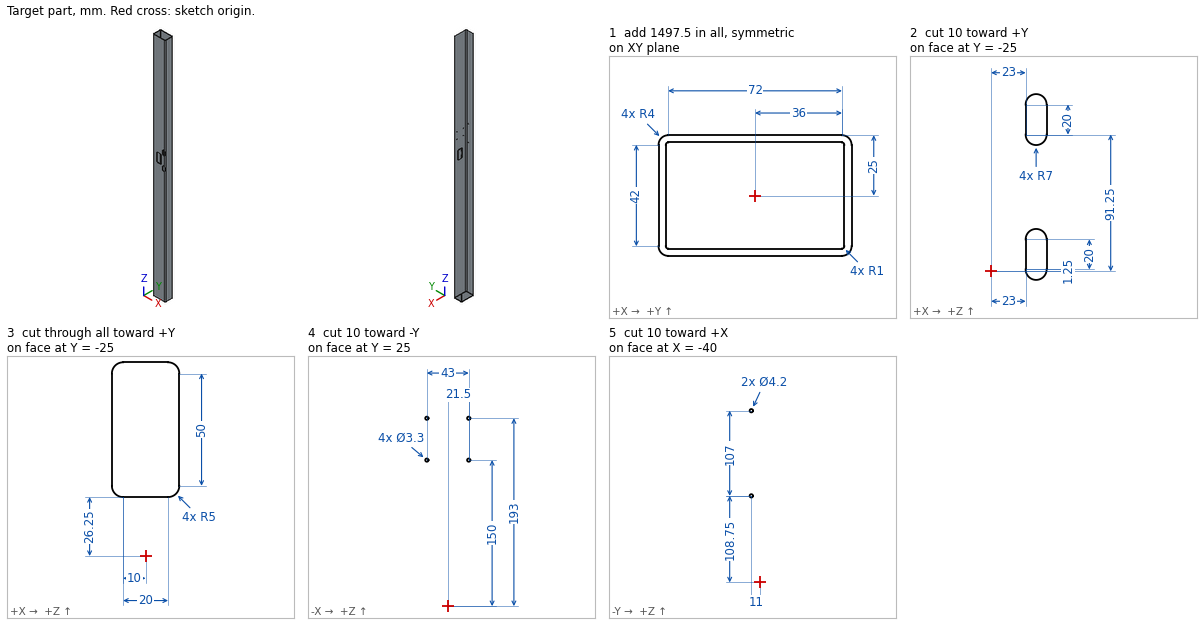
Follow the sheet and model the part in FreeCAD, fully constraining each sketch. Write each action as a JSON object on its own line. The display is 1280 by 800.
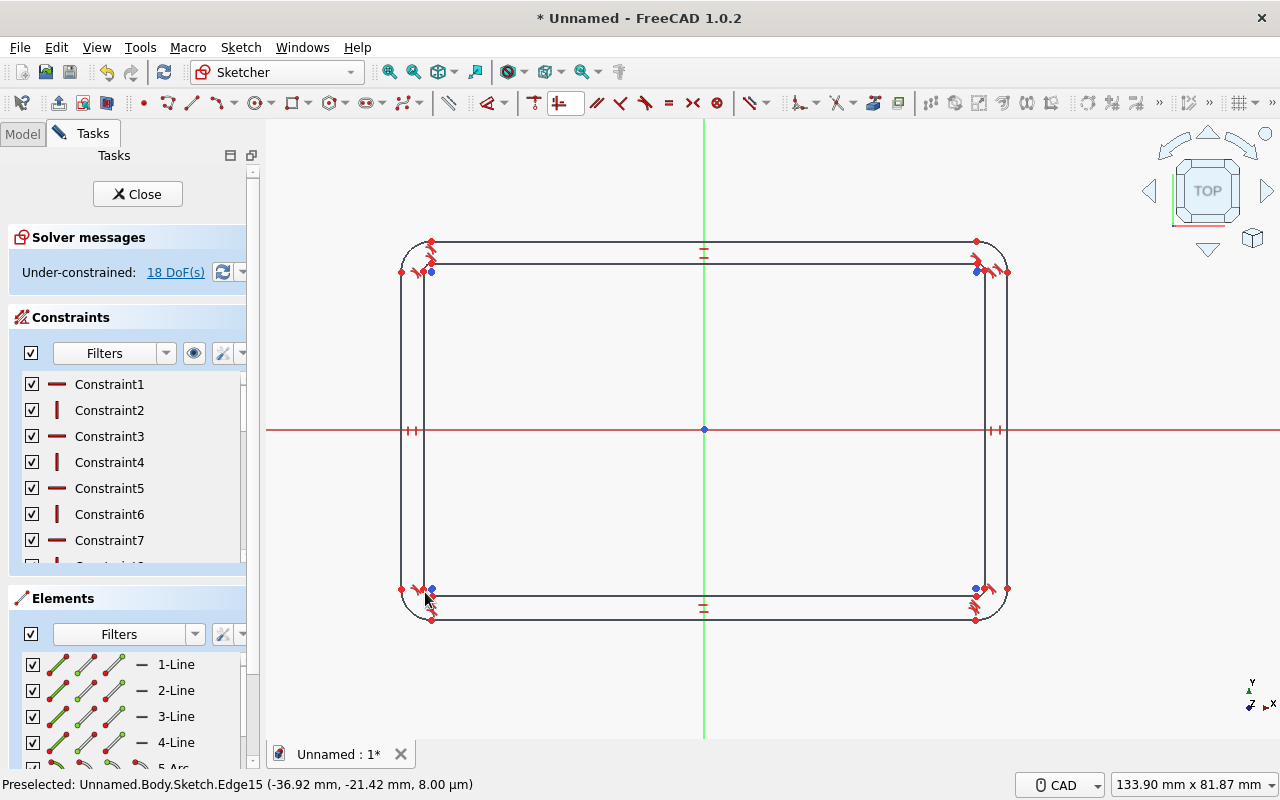
{"action": "left_click", "coordinate": [424, 526]}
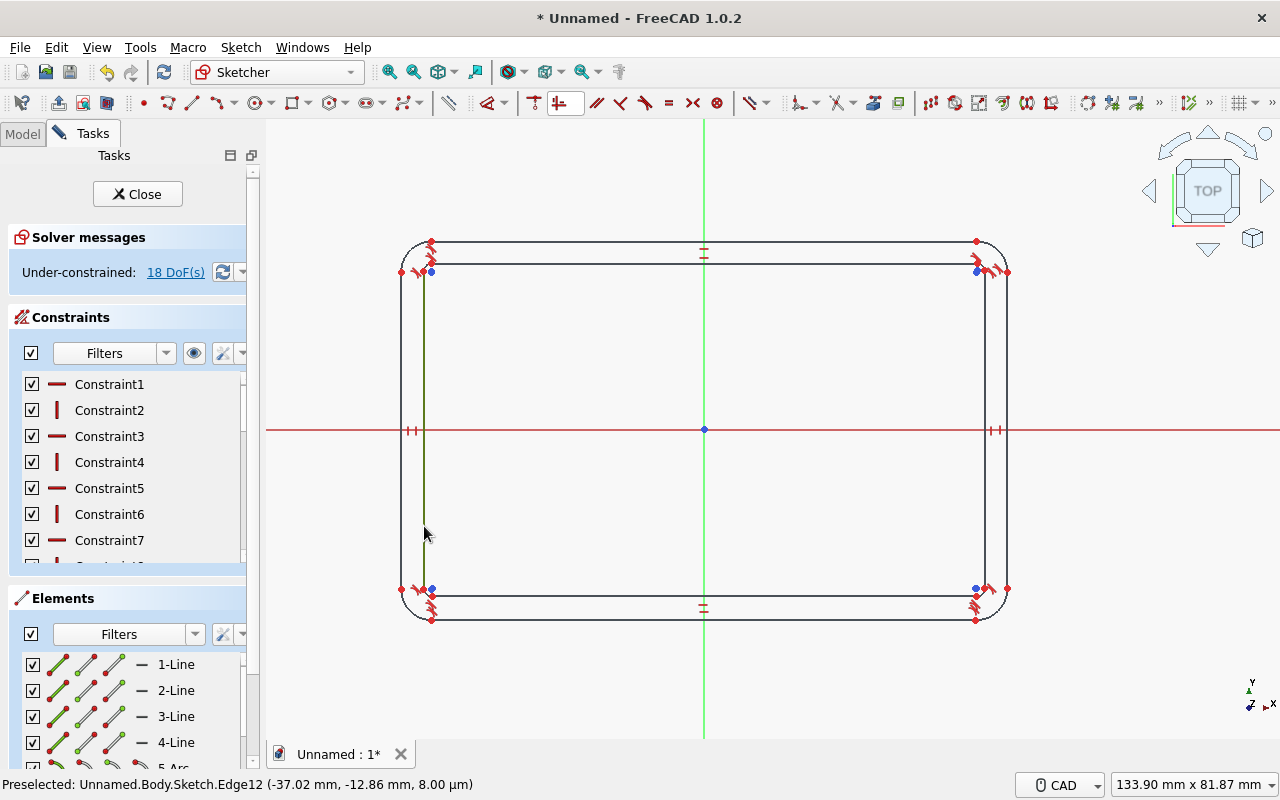
{"action": "scroll", "coordinate": [427, 594], "scroll_direction": "up", "scroll_amount": 5}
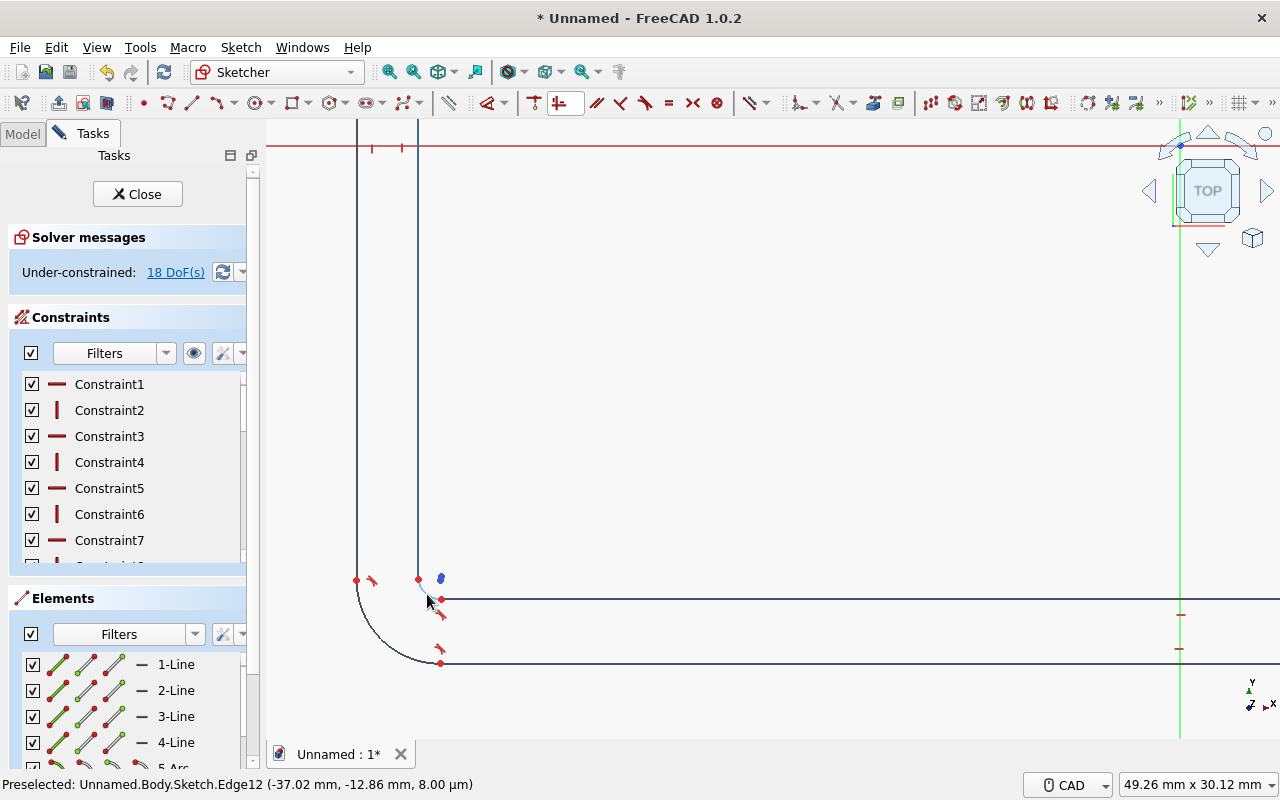
{"action": "left_click", "coordinate": [426, 594]}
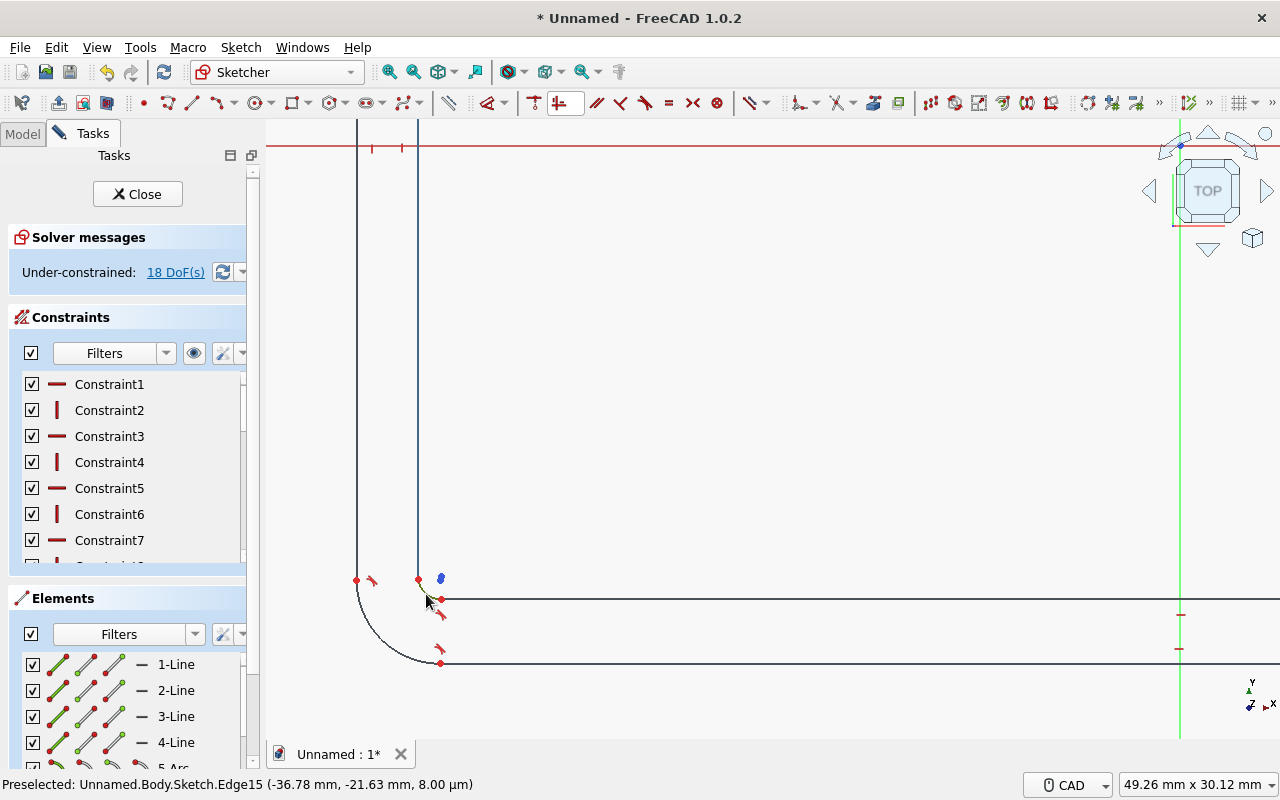
{"action": "key", "text": "t"}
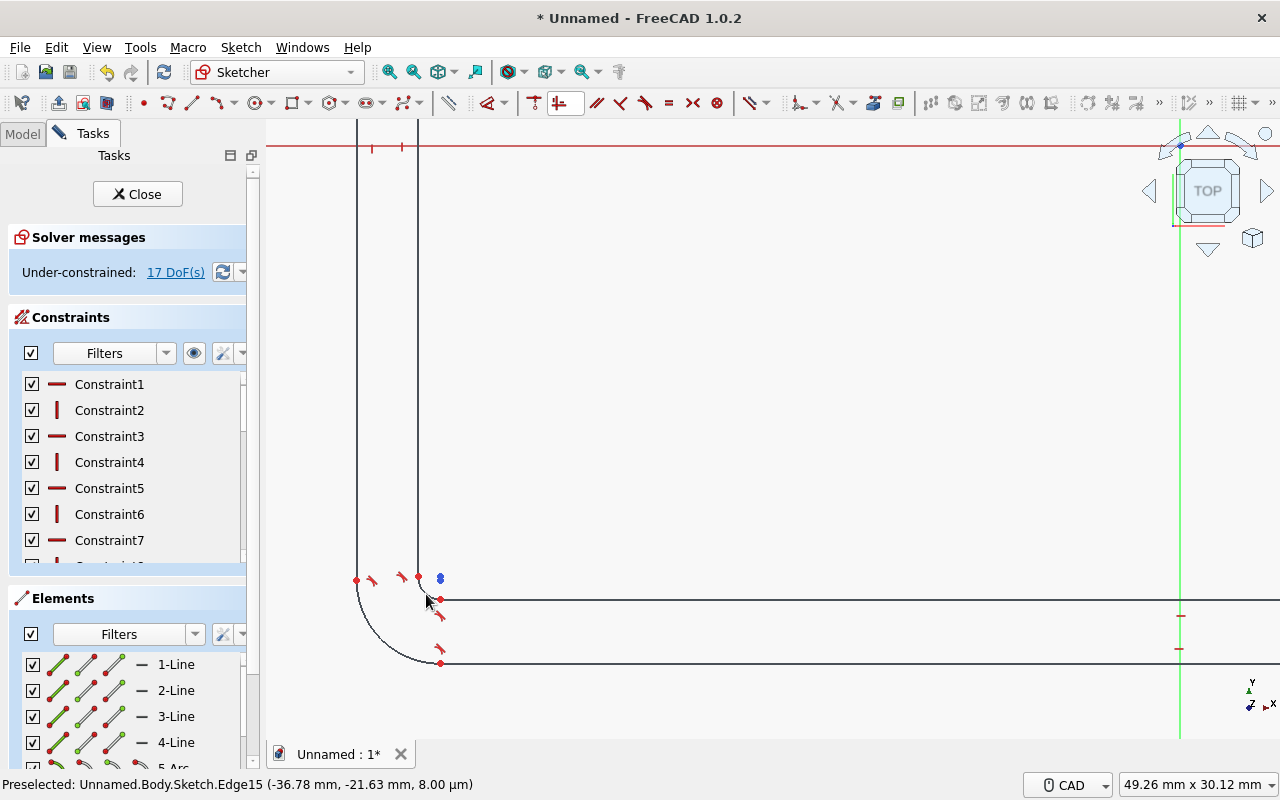
{"action": "left_click", "coordinate": [418, 319]}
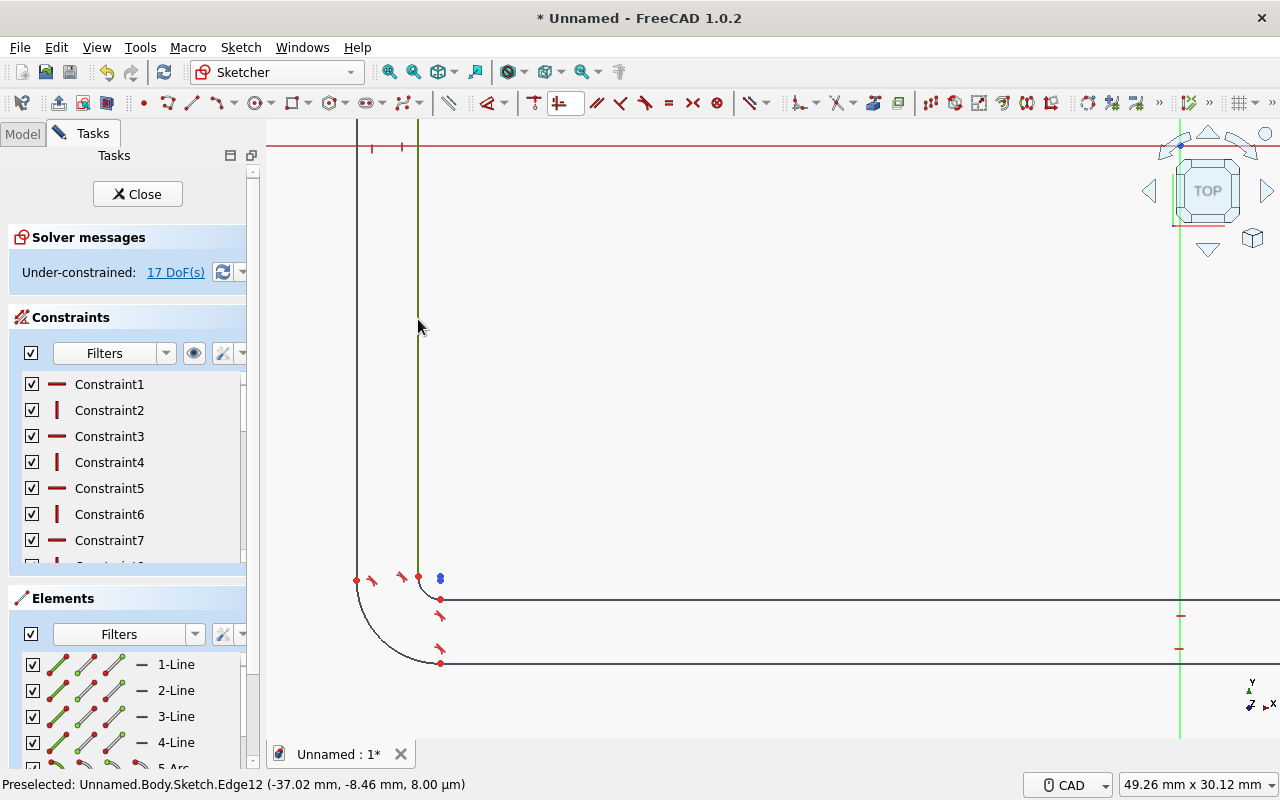
{"action": "scroll", "coordinate": [427, 594], "scroll_direction": "down", "scroll_amount": 5}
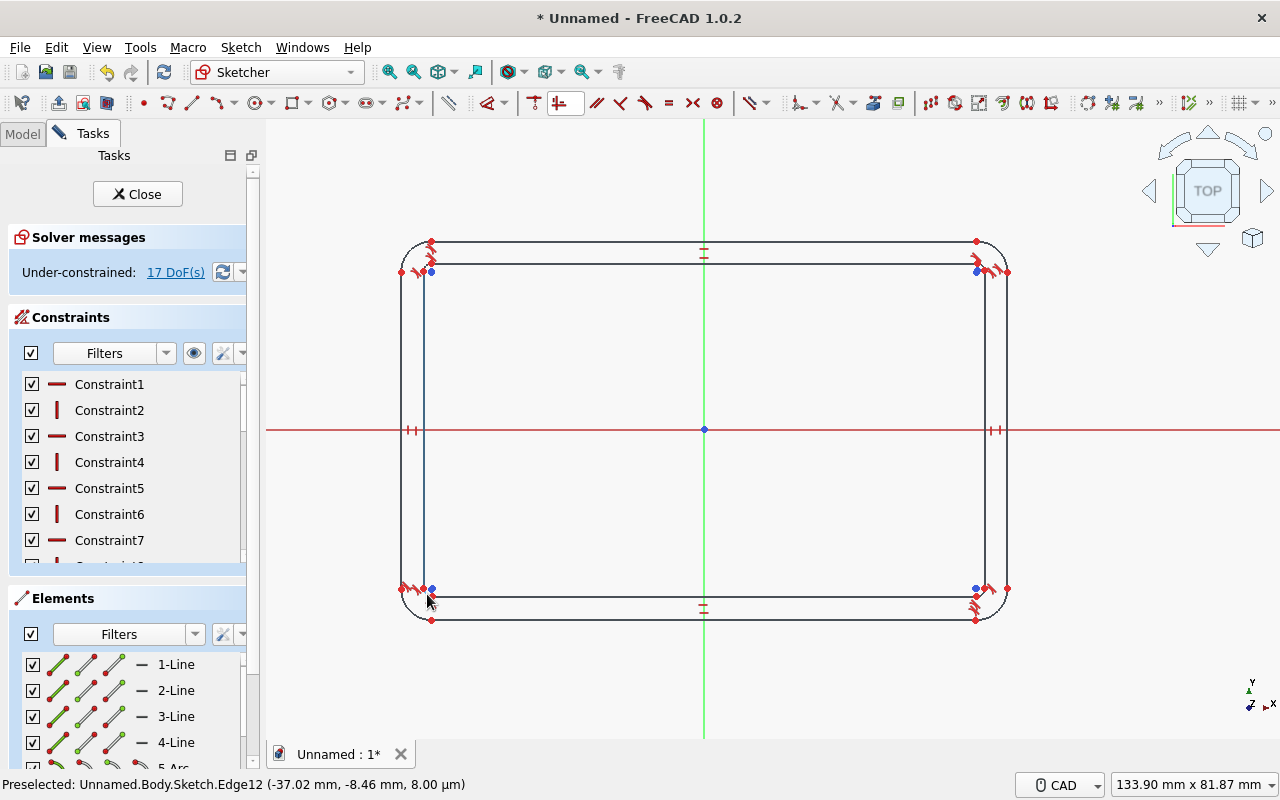
{"action": "scroll", "coordinate": [428, 264], "scroll_direction": "up", "scroll_amount": 7}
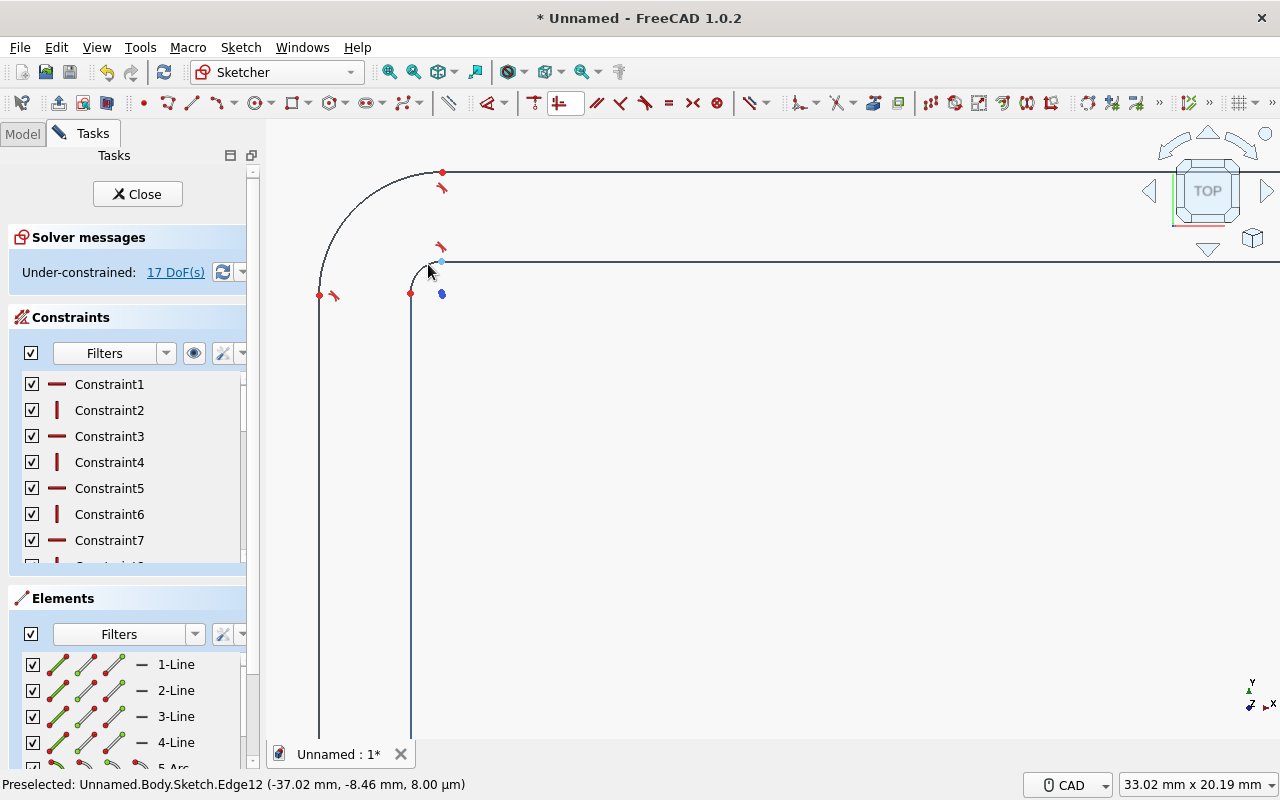
{"action": "left_click", "coordinate": [427, 265]}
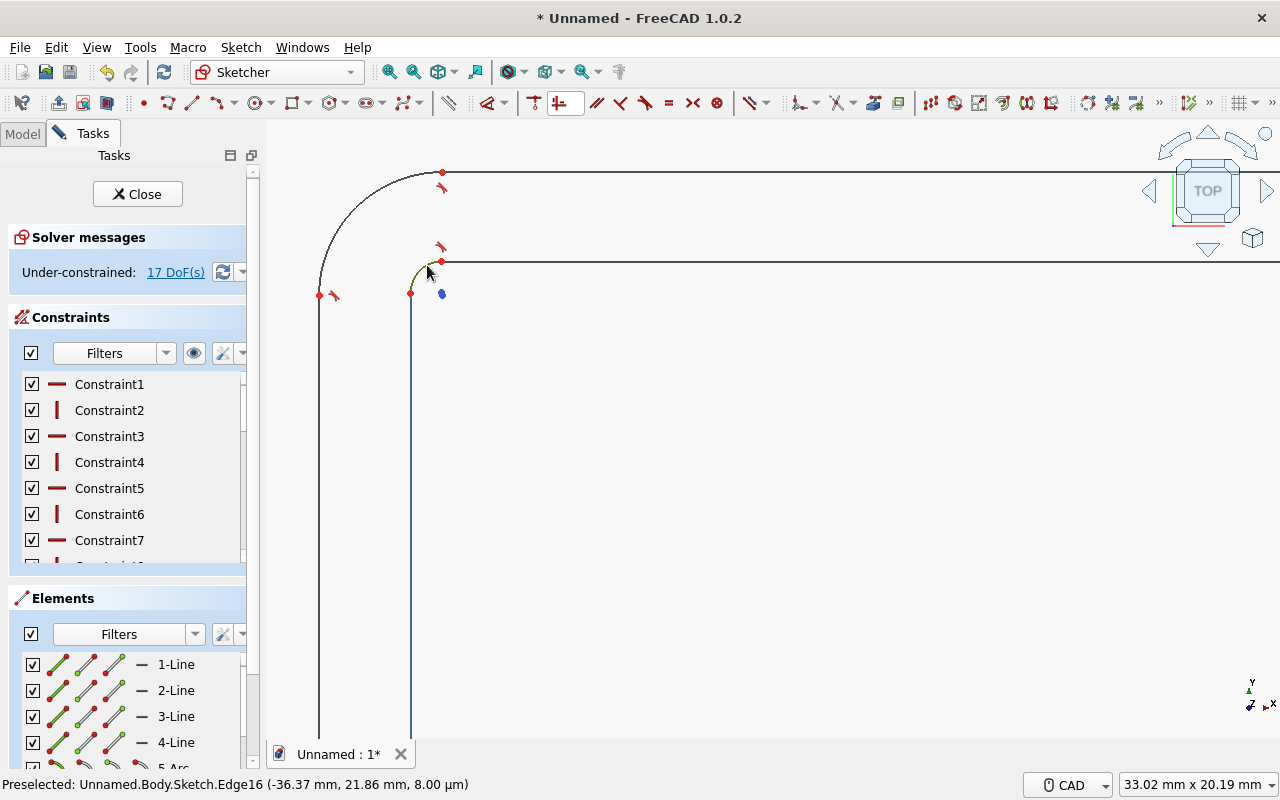
{"action": "key", "text": "t"}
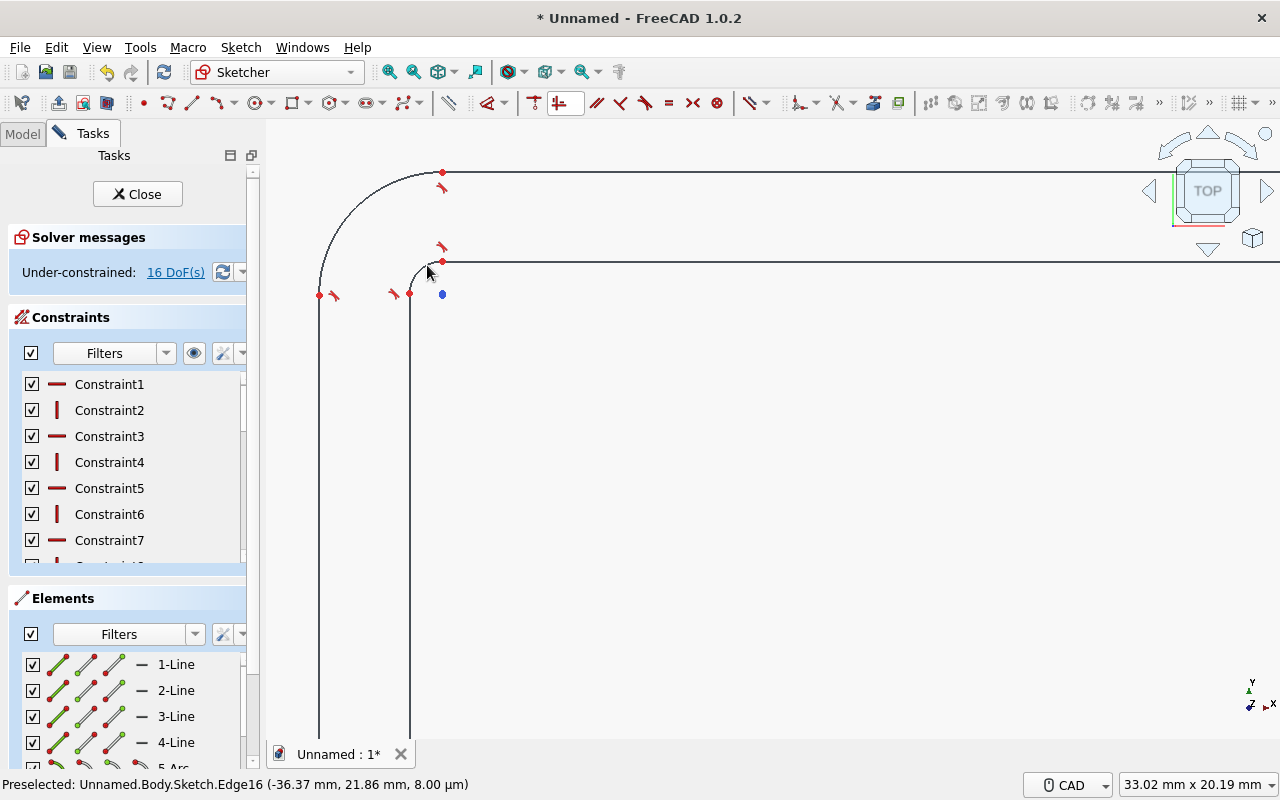
{"action": "scroll", "coordinate": [428, 263], "scroll_direction": "down", "scroll_amount": 7}